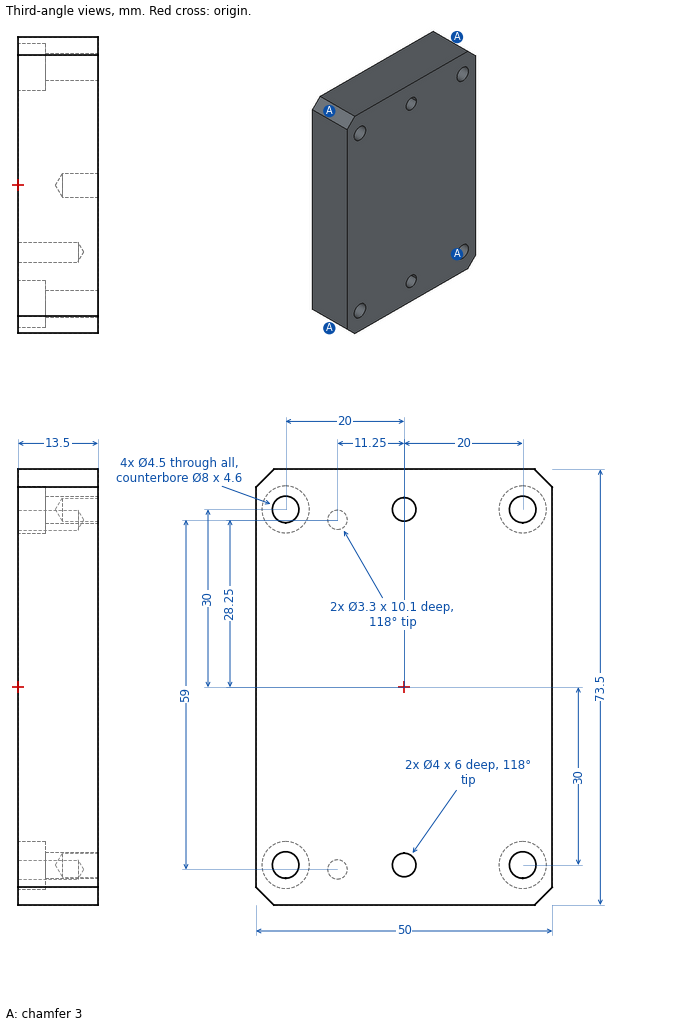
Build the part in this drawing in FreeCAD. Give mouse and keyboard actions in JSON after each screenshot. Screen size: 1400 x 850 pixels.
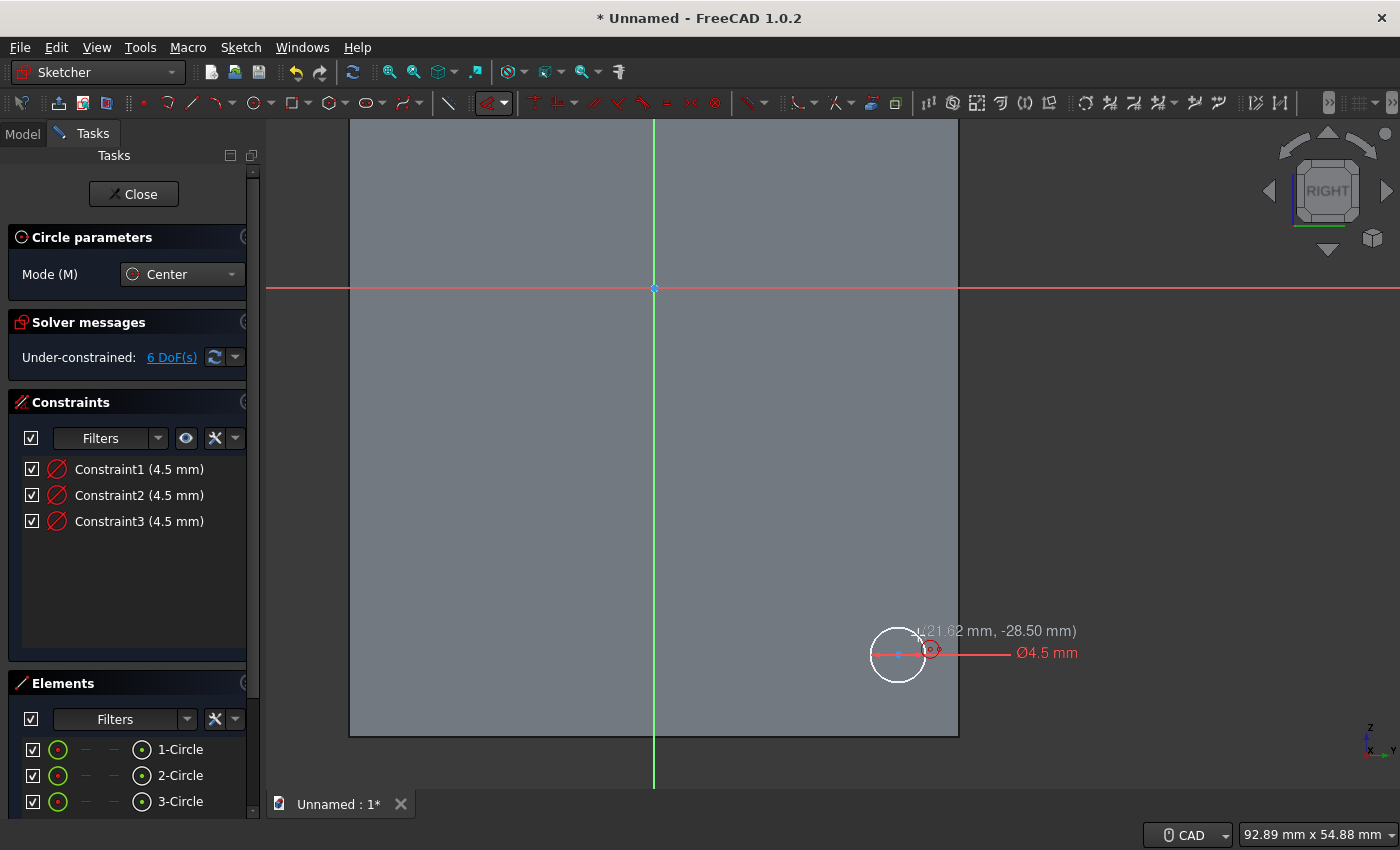
{"action": "left_click", "coordinate": [410, 654]}
{"action": "mouse_move", "coordinate": [429, 635]}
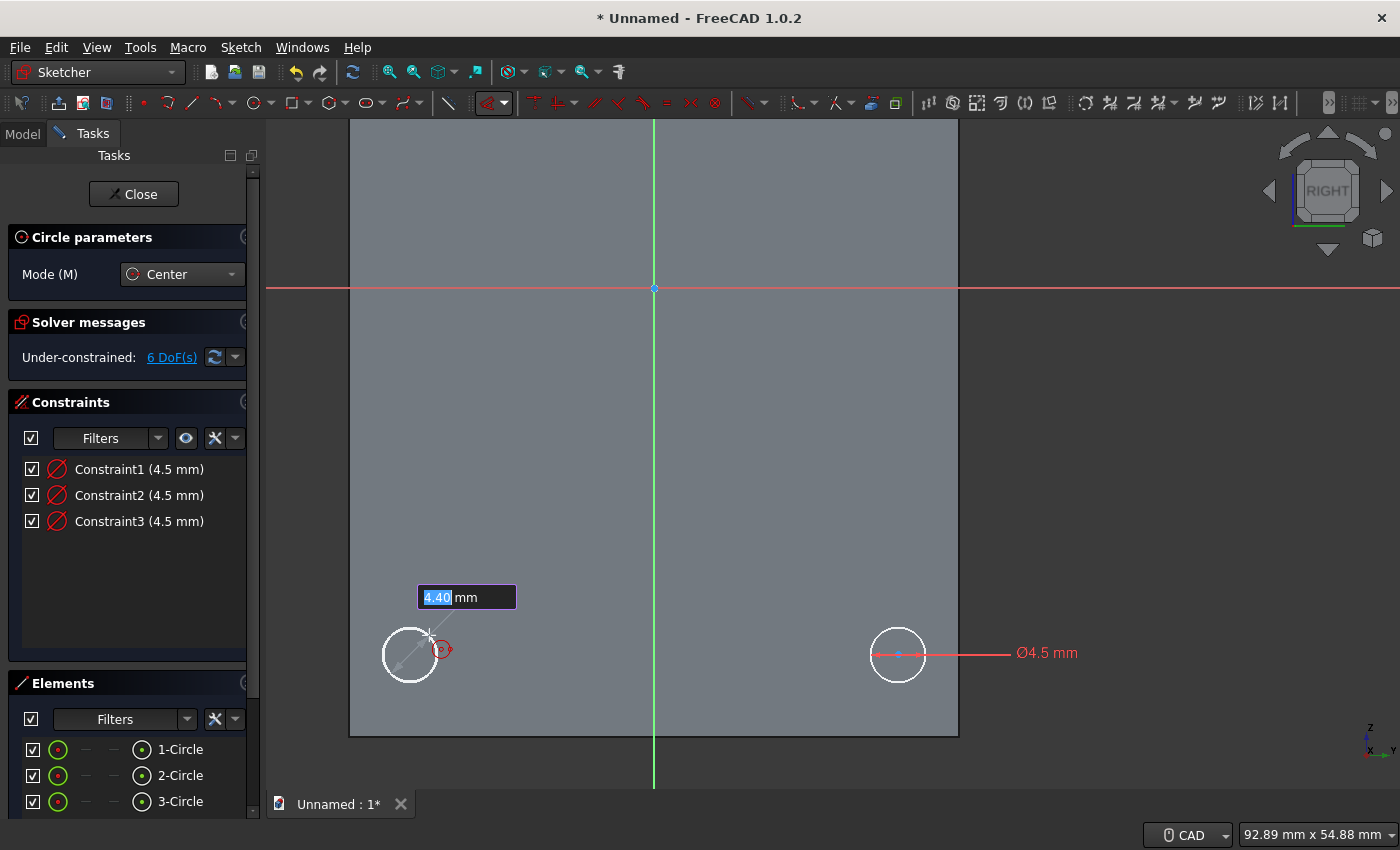
{"action": "type", "text": "4.5"}
{"action": "key", "text": "Return"}
{"action": "key", "text": "Escape"}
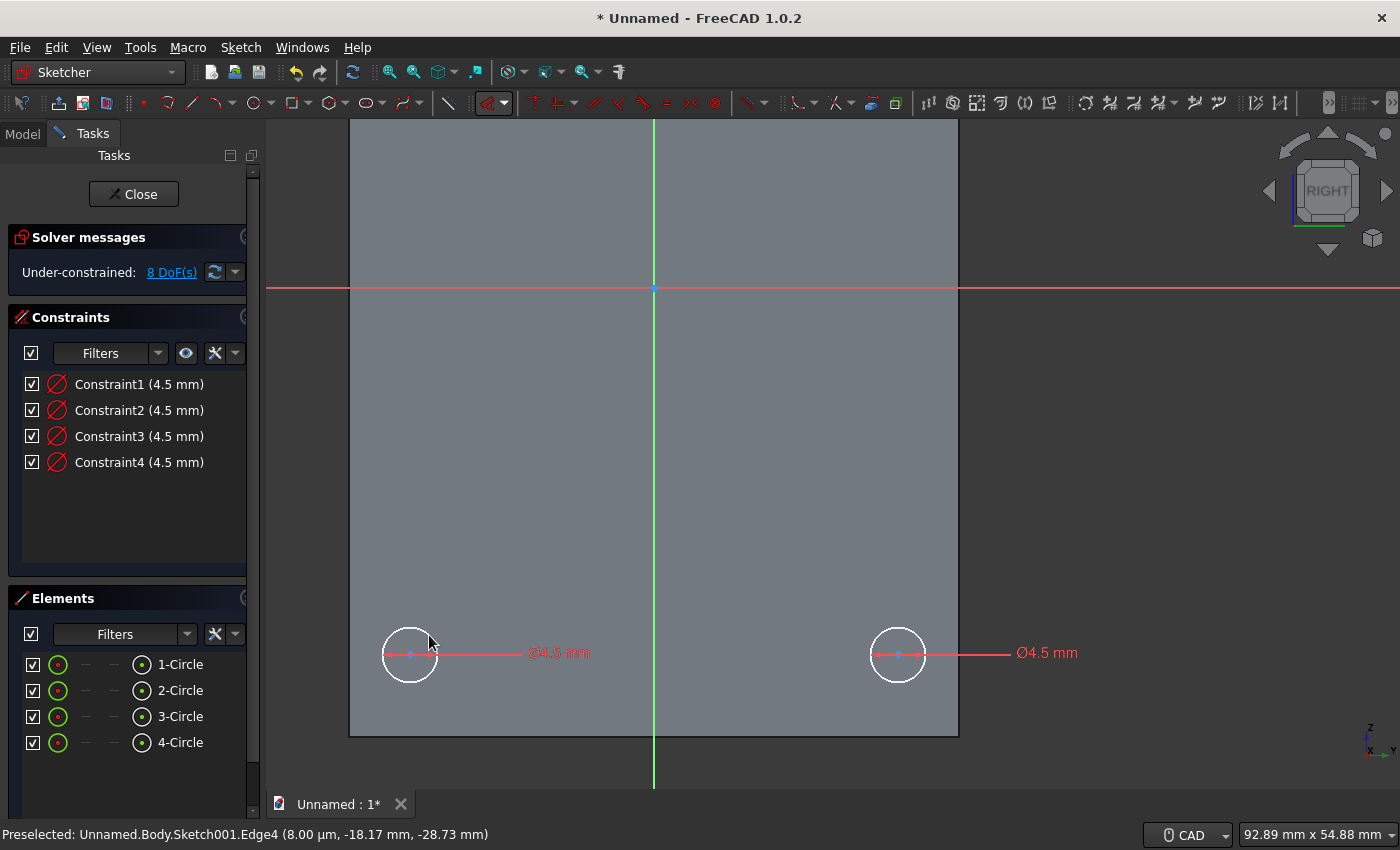
{"action": "scroll", "coordinate": [899, 656], "scroll_direction": "down", "scroll_amount": 3}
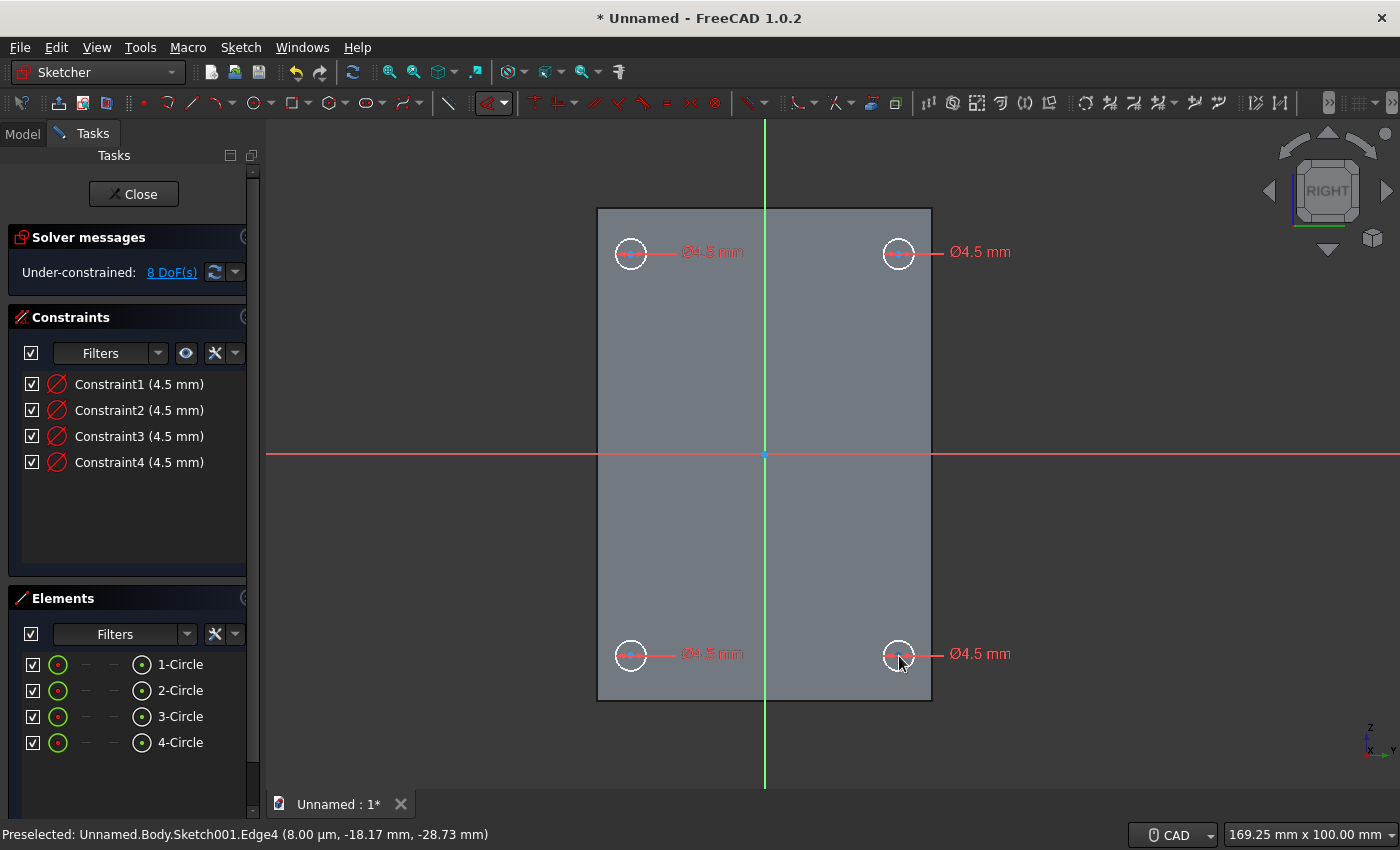
{"action": "left_click", "coordinate": [631, 254]}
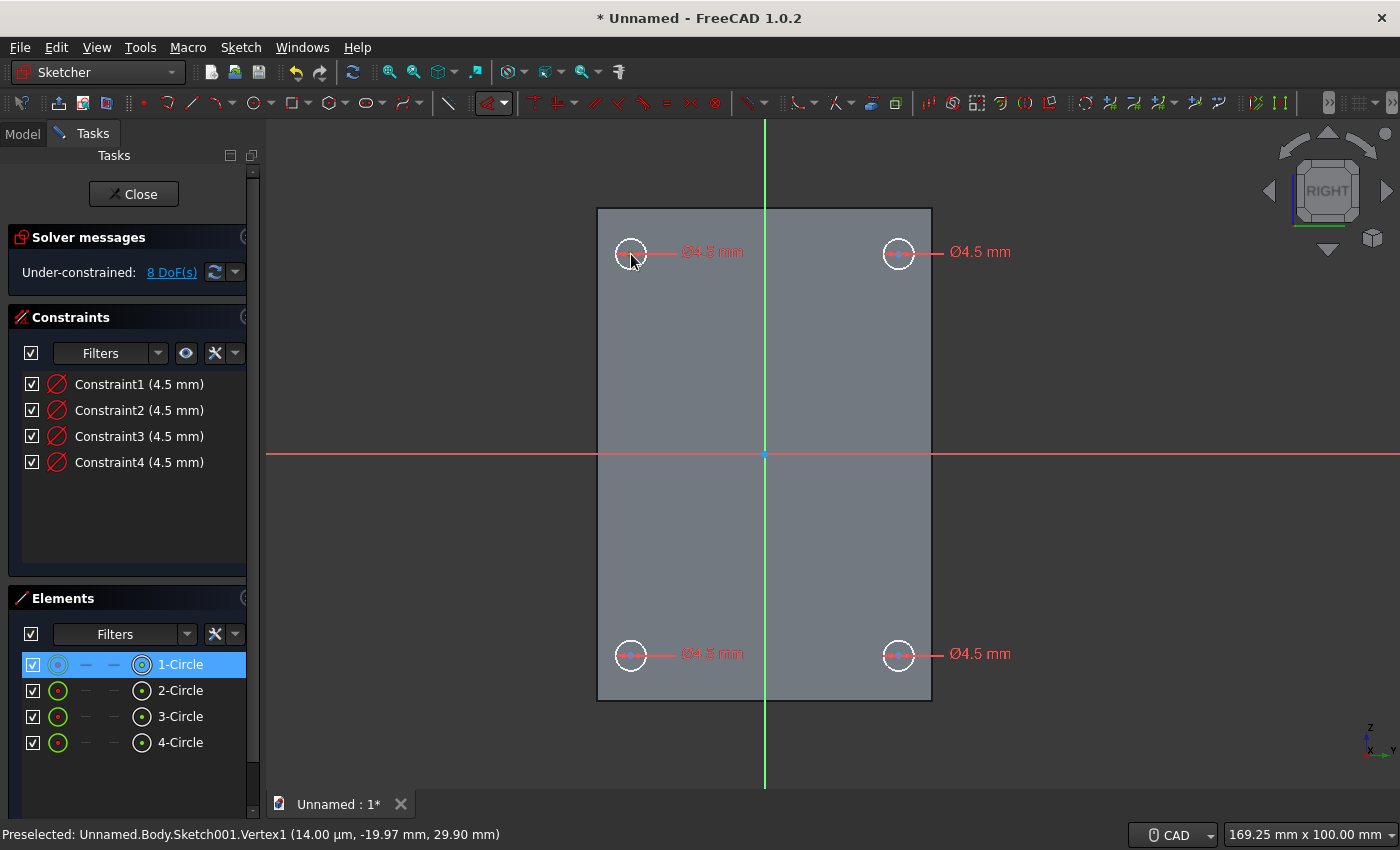
{"action": "left_click", "coordinate": [899, 254]}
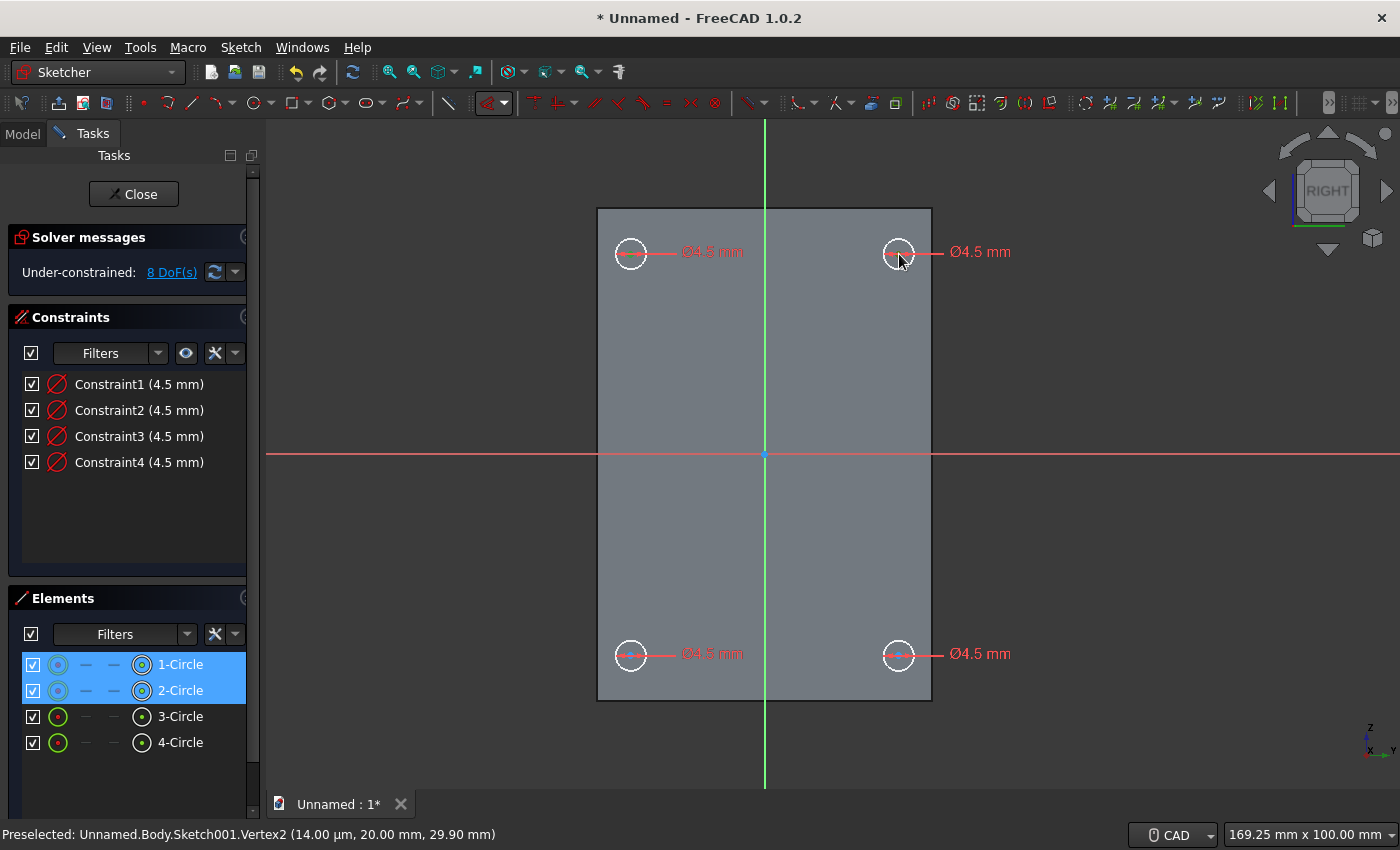
{"action": "left_click", "coordinate": [576, 104]}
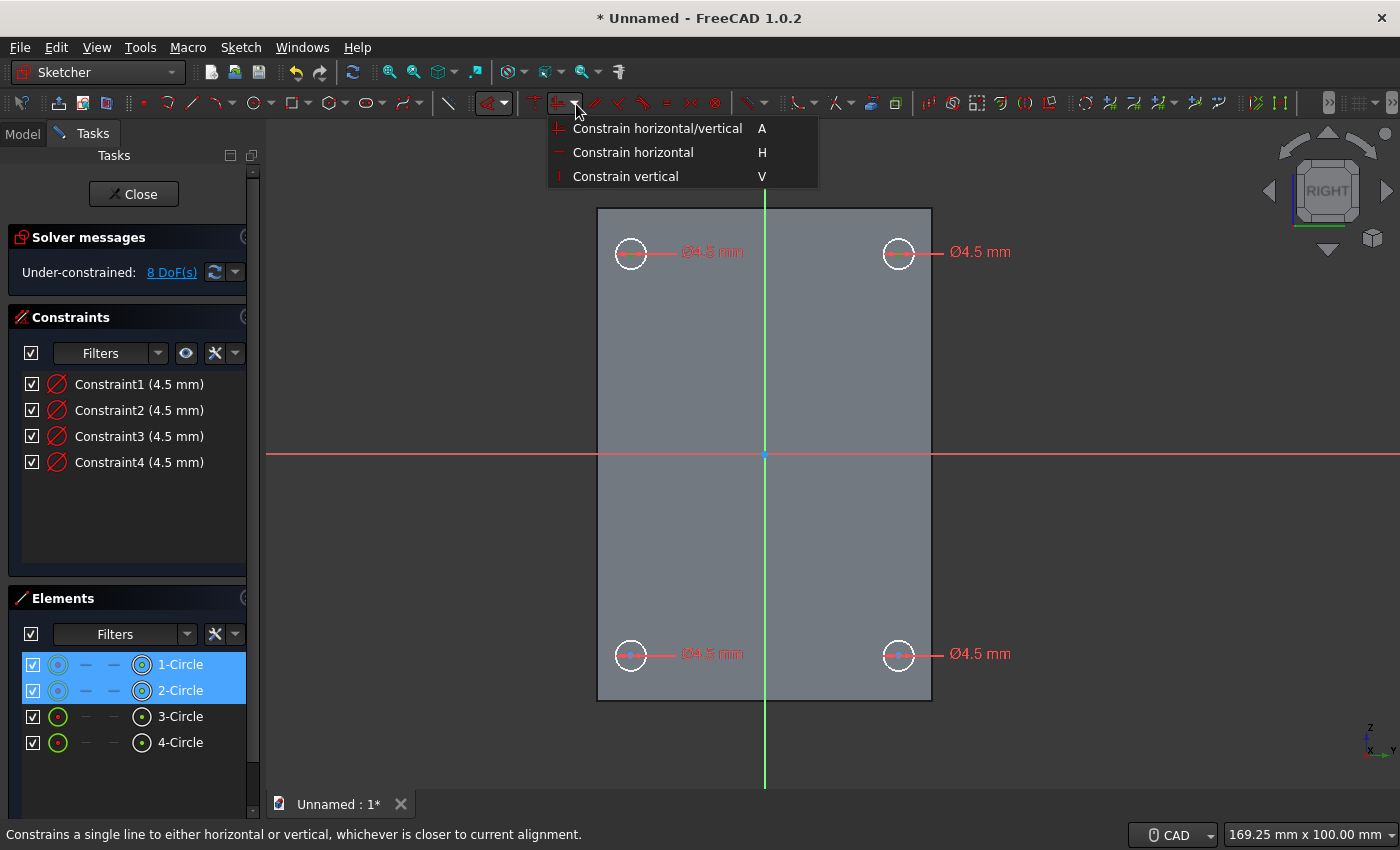
{"action": "left_click", "coordinate": [683, 152]}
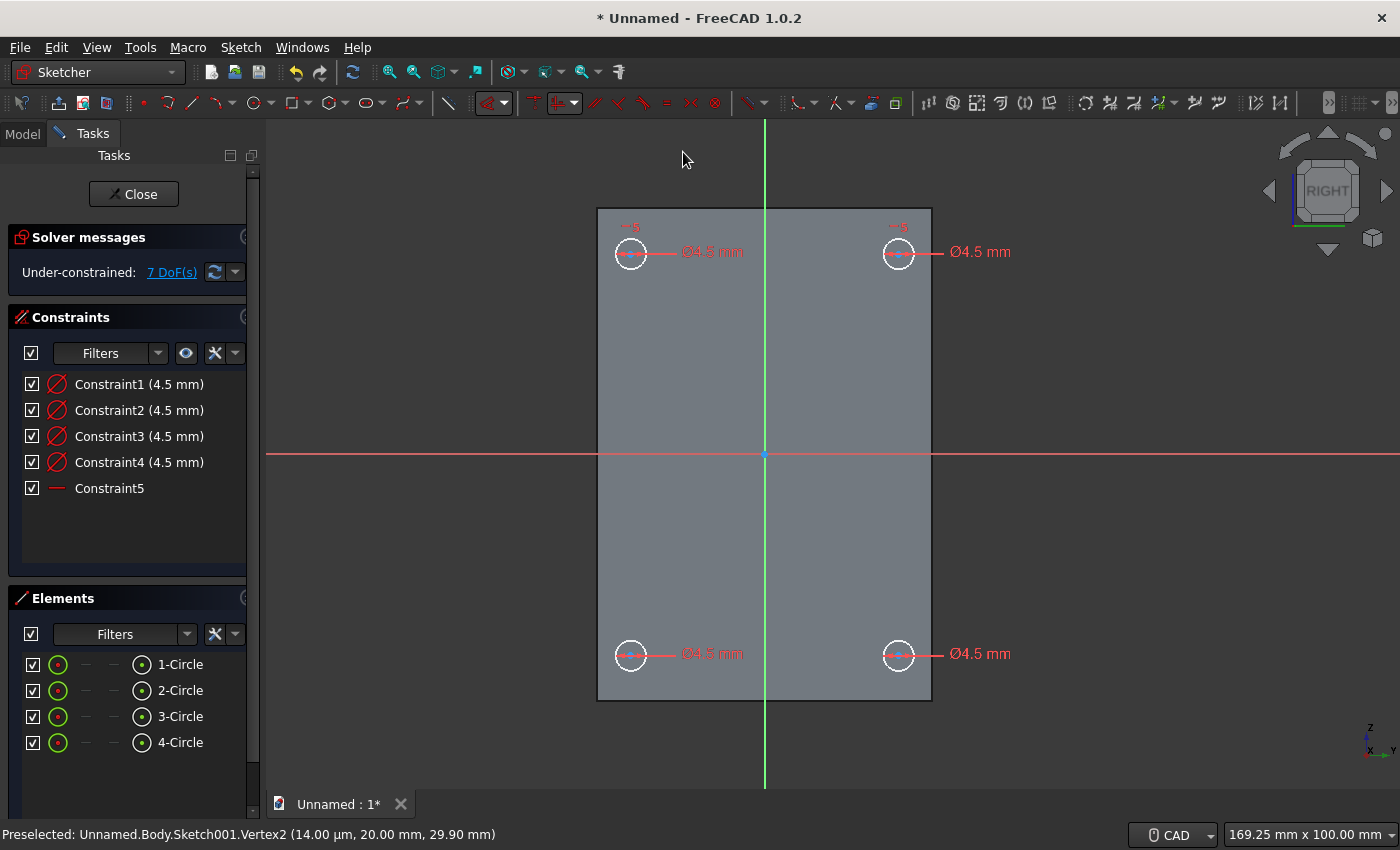
{"action": "left_click", "coordinate": [899, 254]}